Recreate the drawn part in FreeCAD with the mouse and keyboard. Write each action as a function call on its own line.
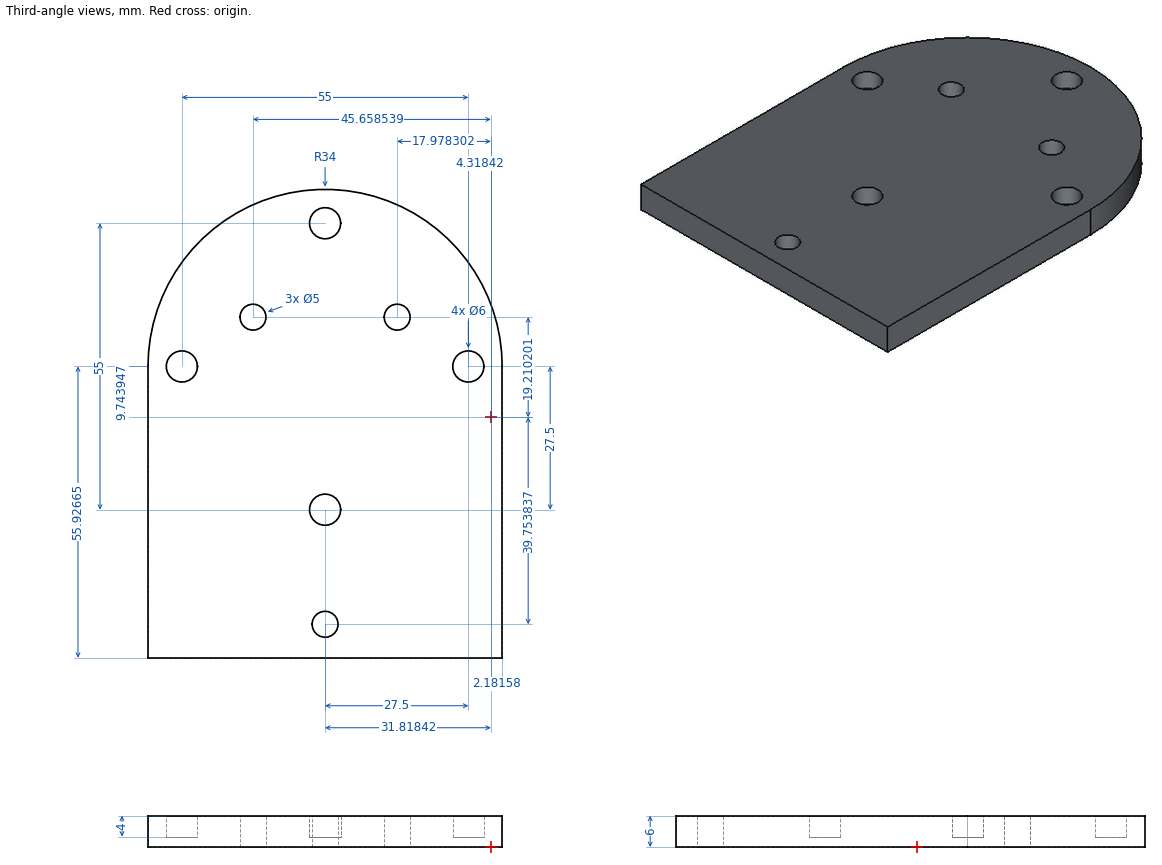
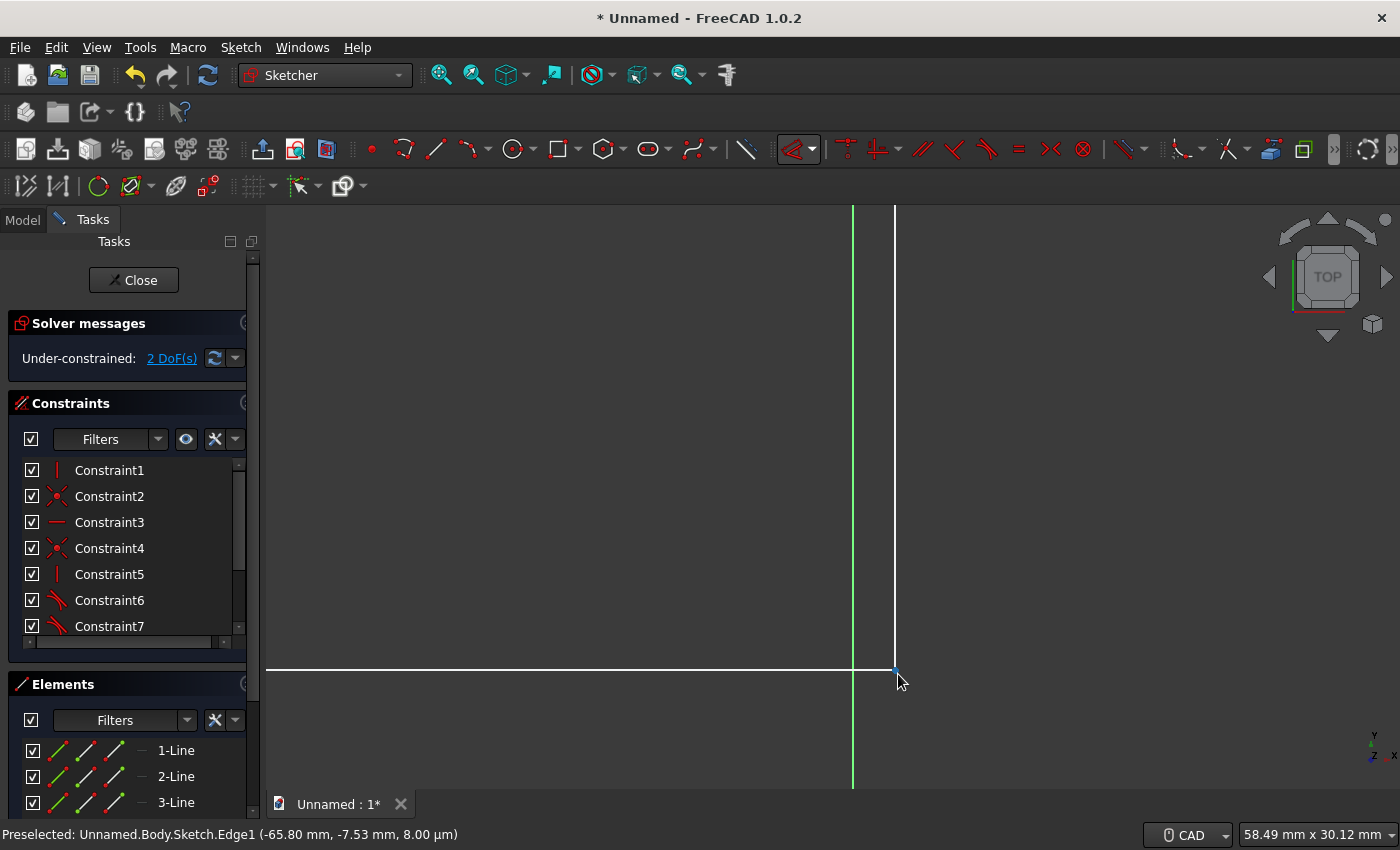
click(895, 670)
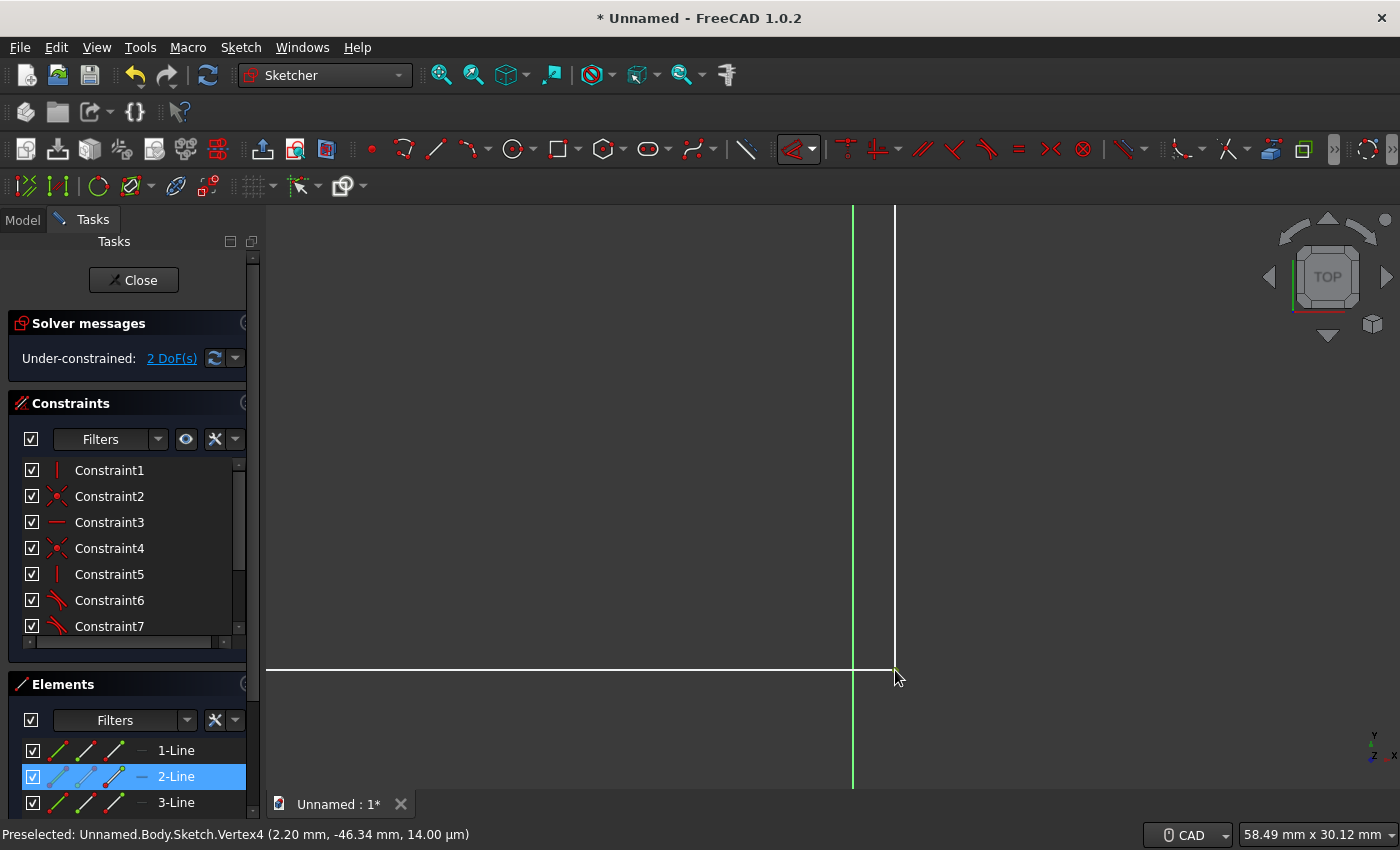
key(l)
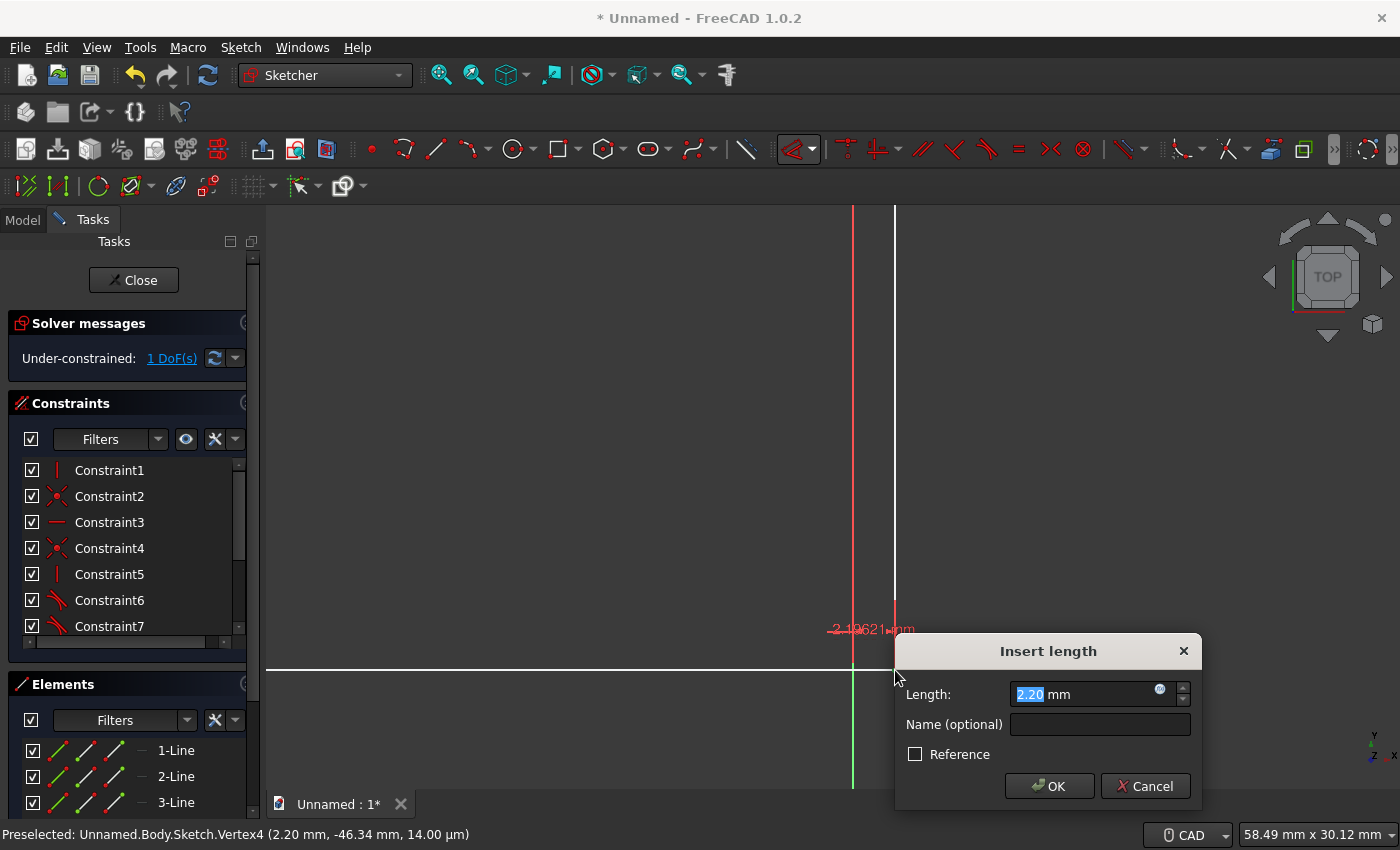
text(2.18158)
key(Return)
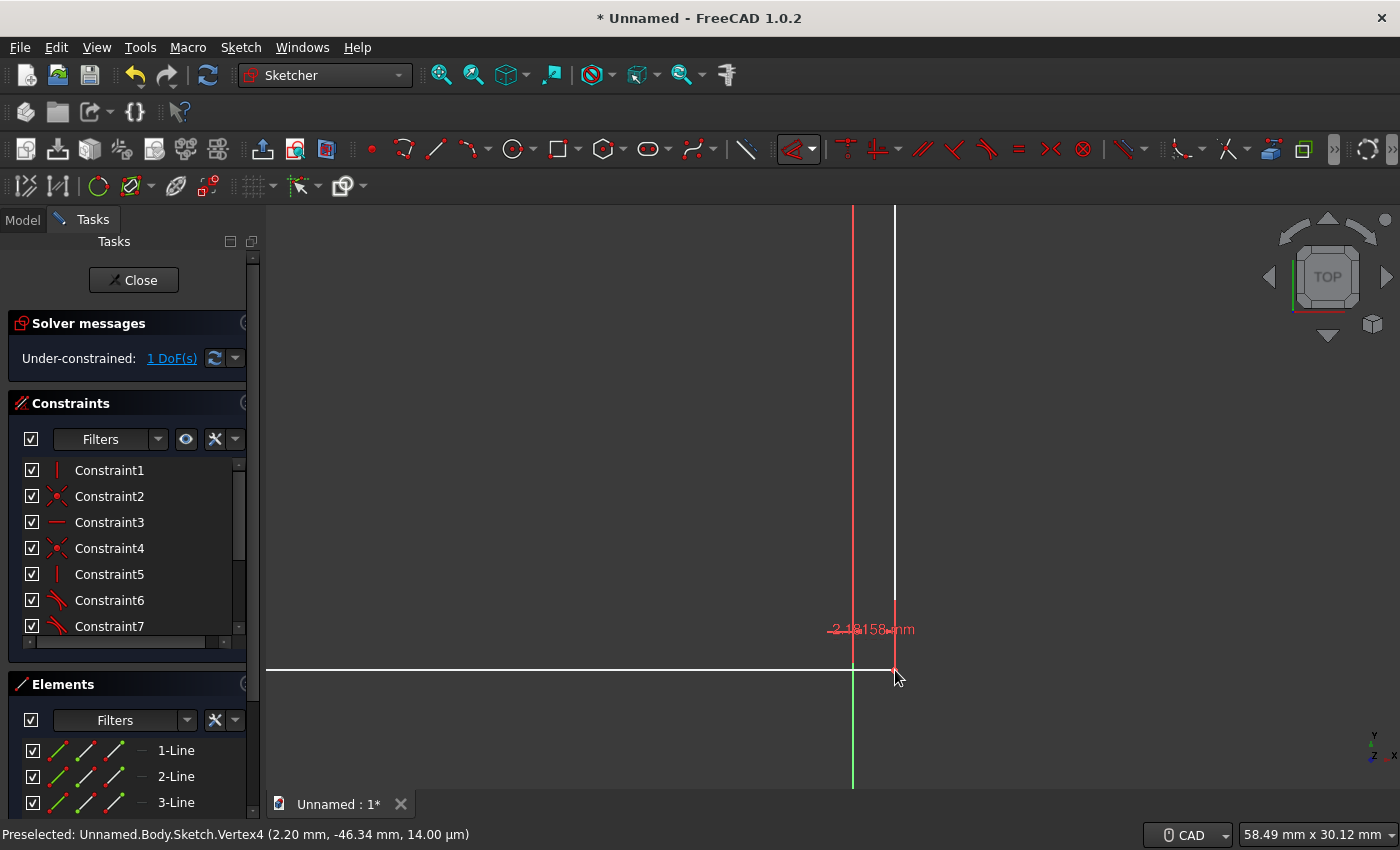
scroll(898, 674, down, 8)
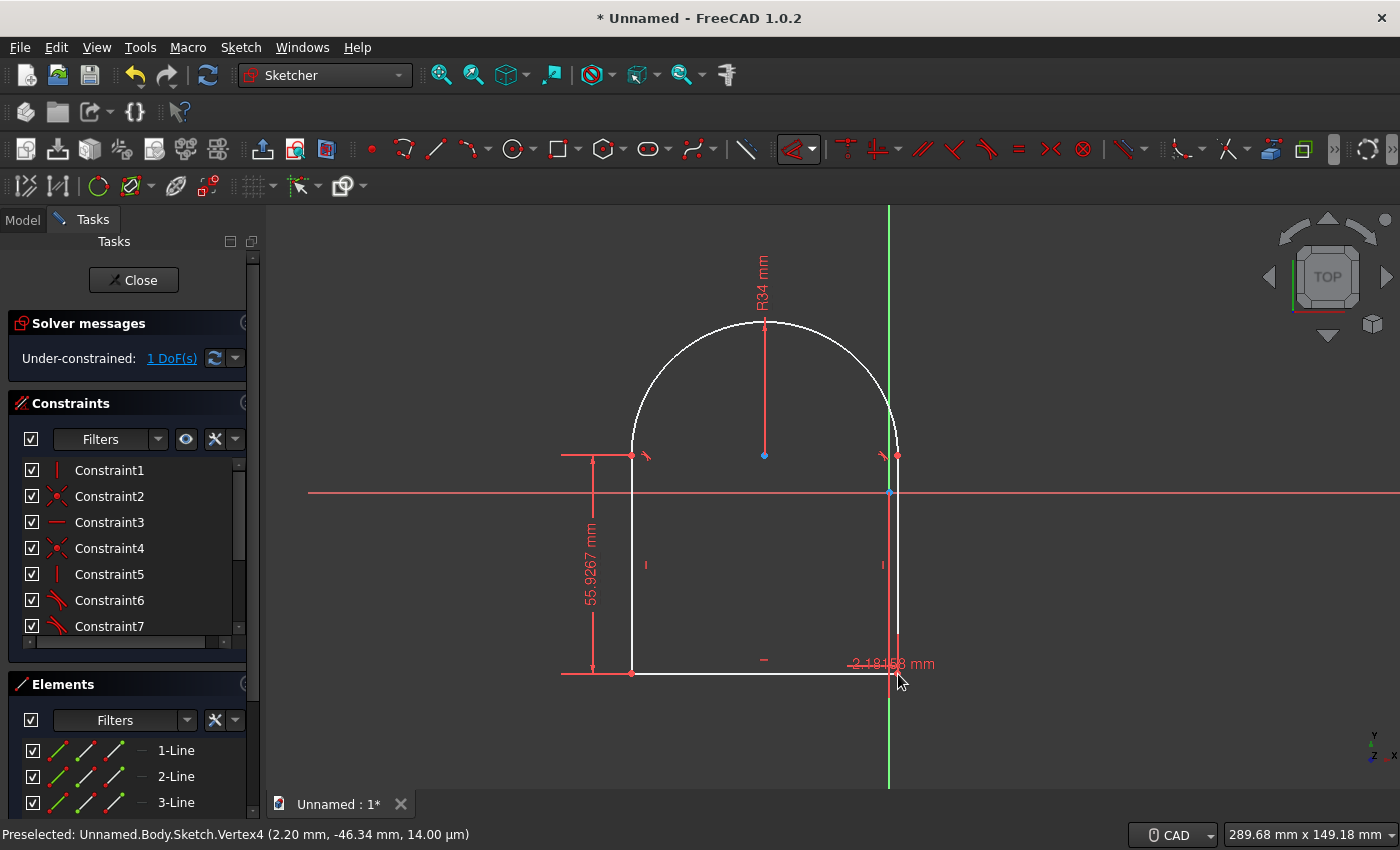
click(632, 455)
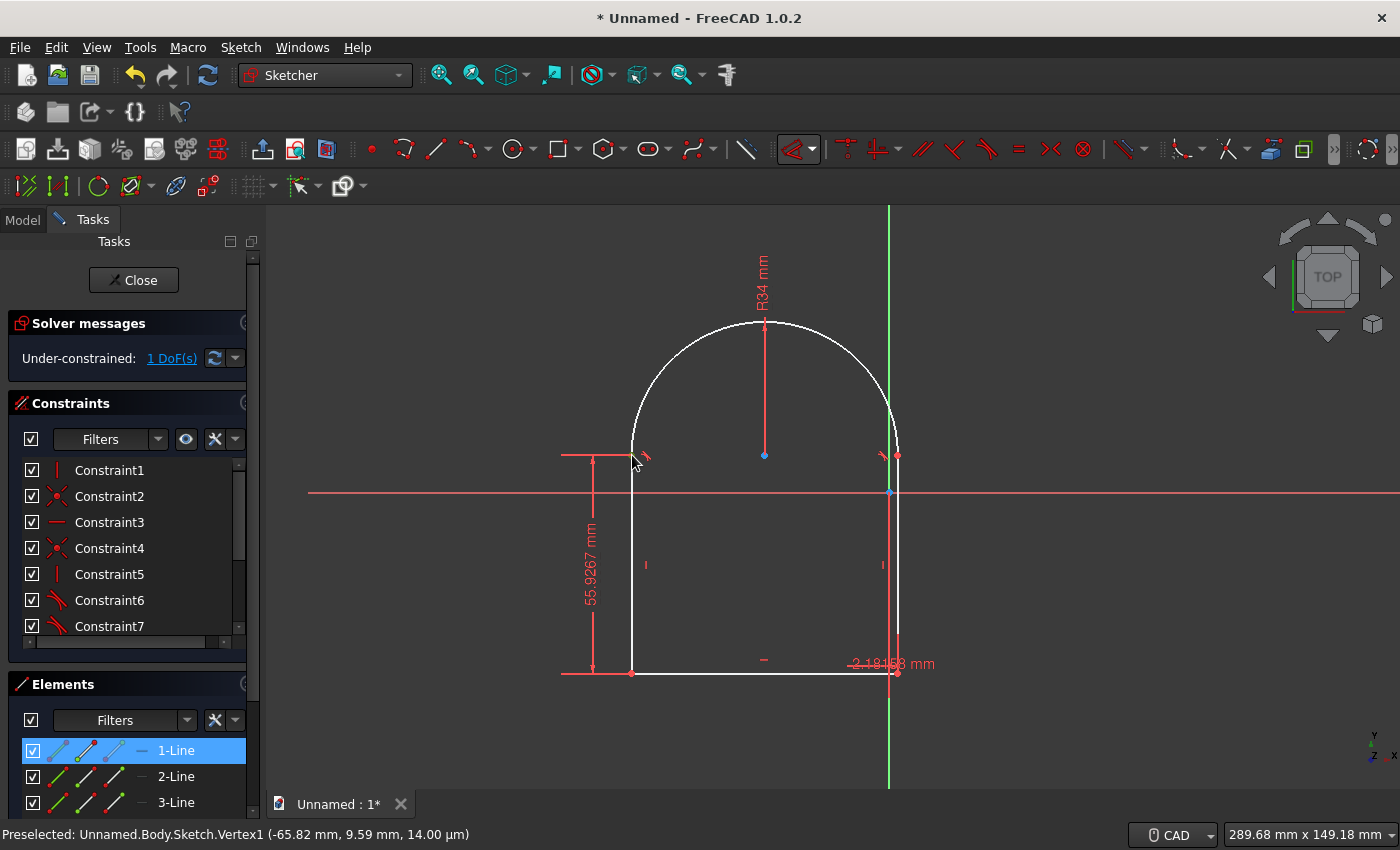
key(i)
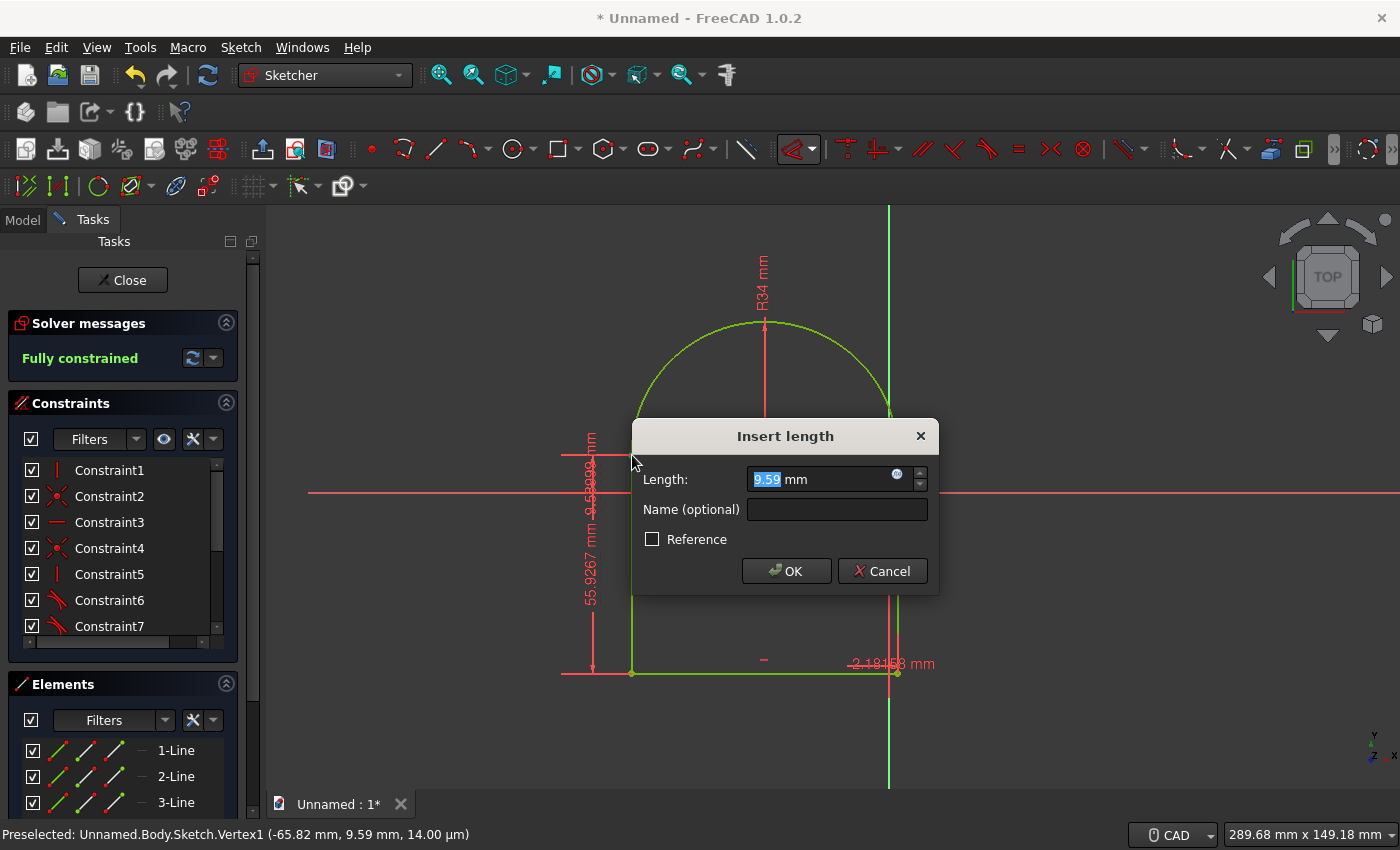
text(9.743947)
key(Return)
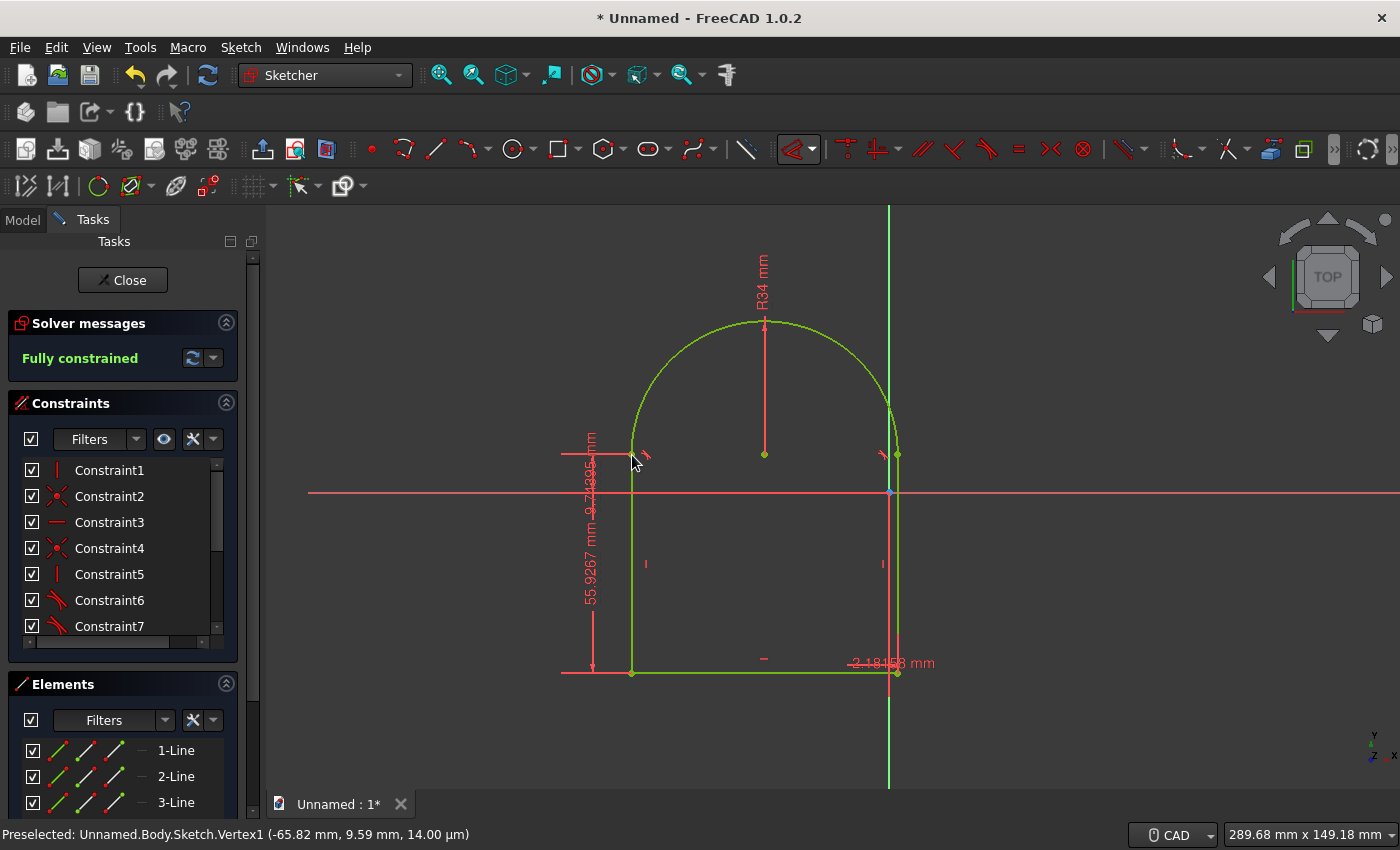
click(123, 280)